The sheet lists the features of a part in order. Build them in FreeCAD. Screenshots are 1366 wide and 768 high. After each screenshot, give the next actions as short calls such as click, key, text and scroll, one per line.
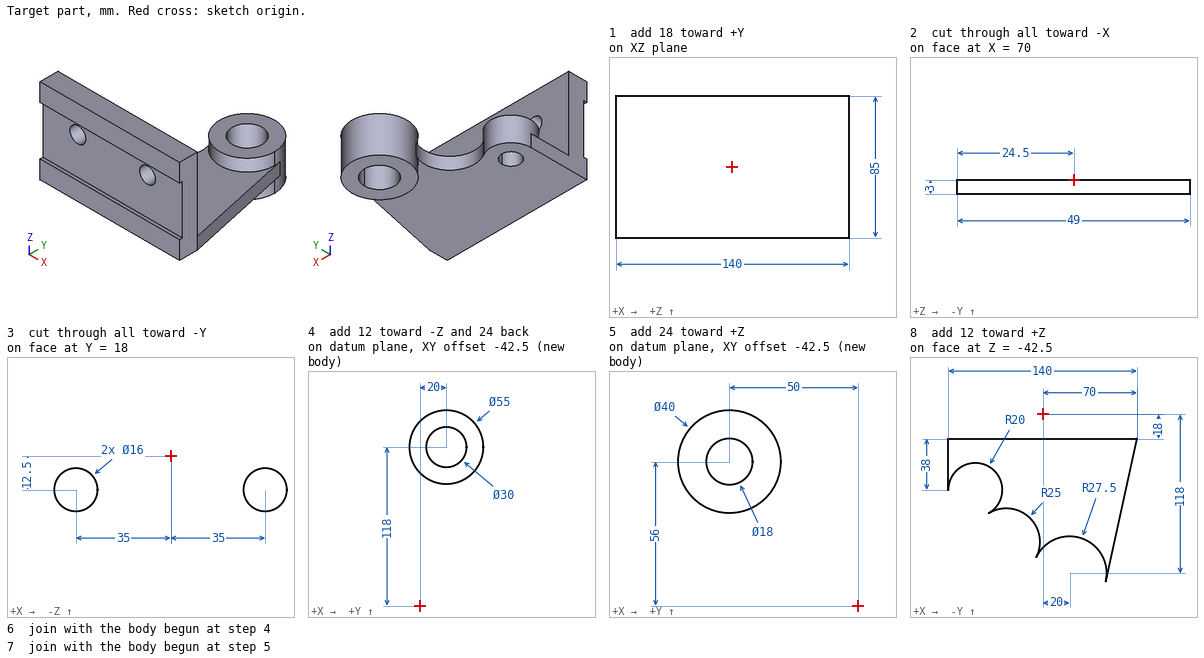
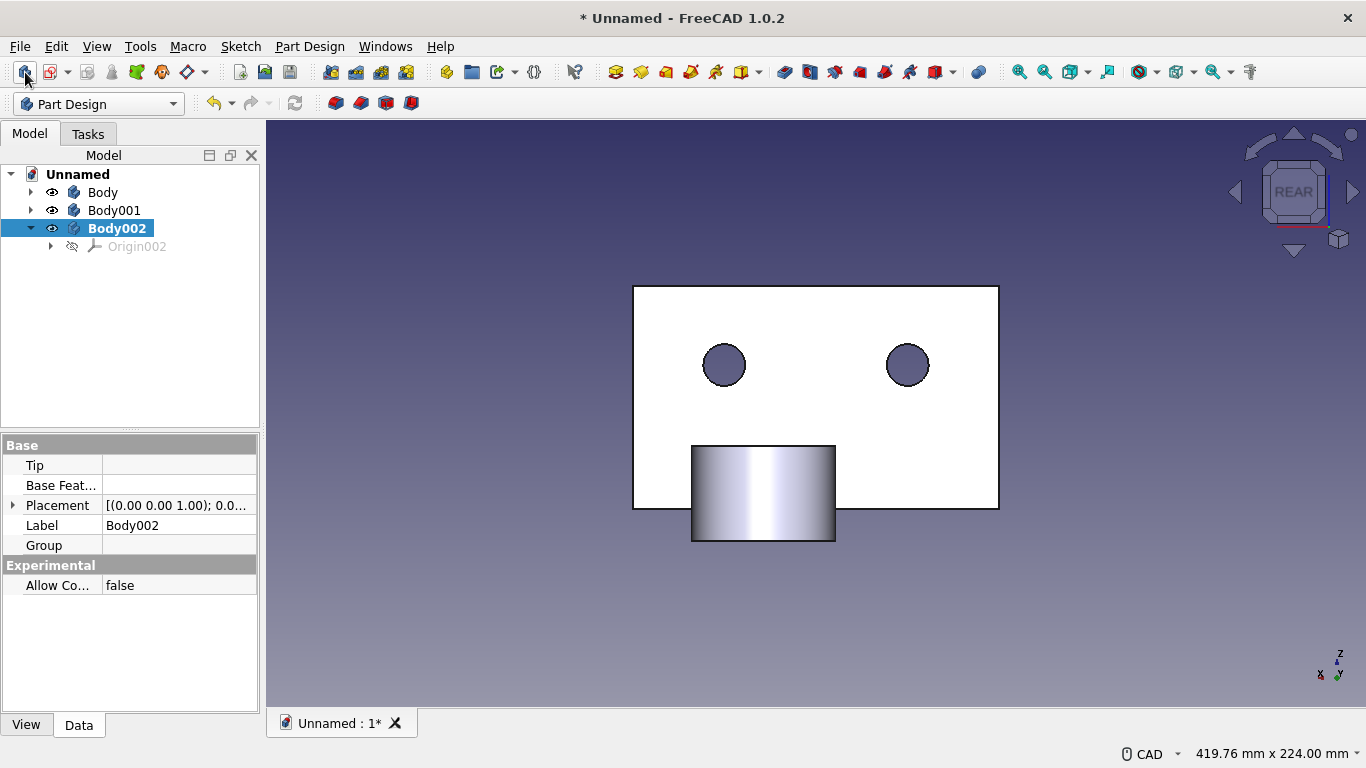
click(51, 246)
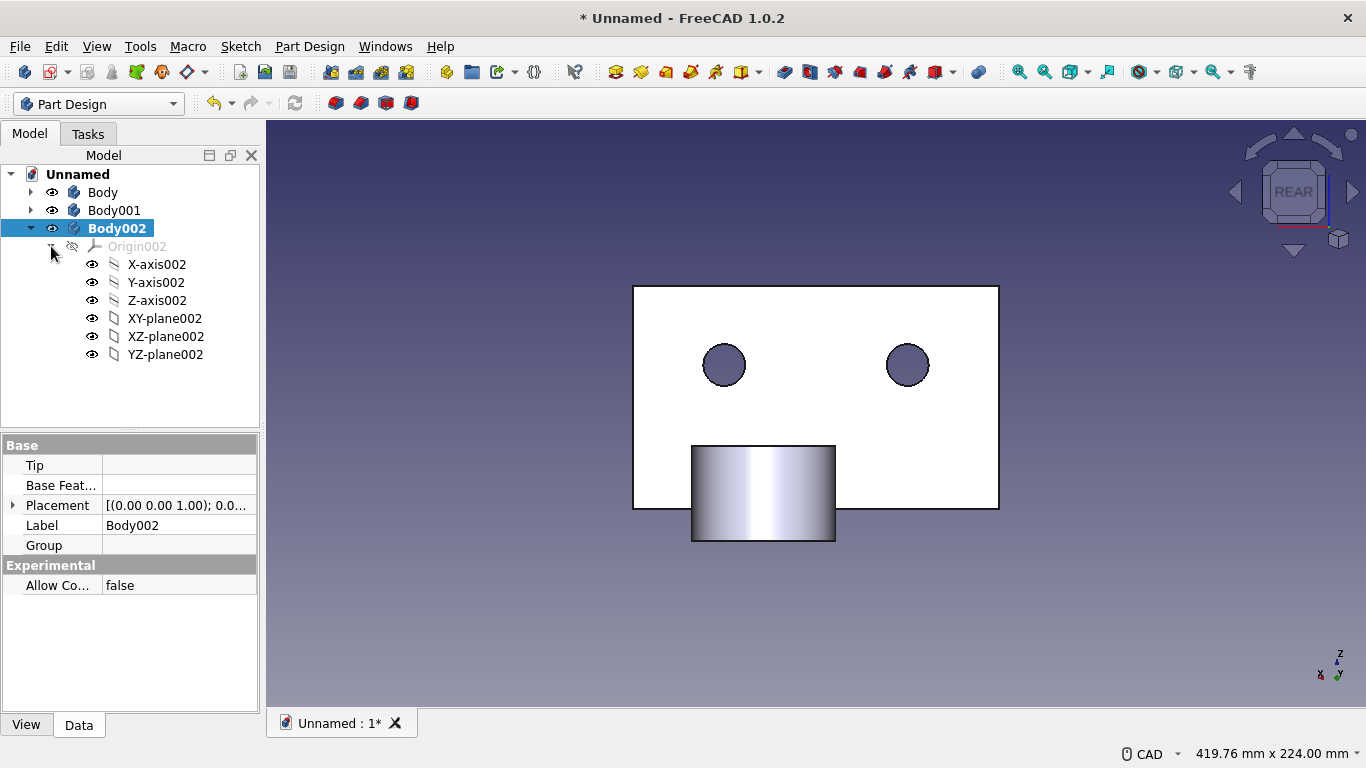
click(137, 318)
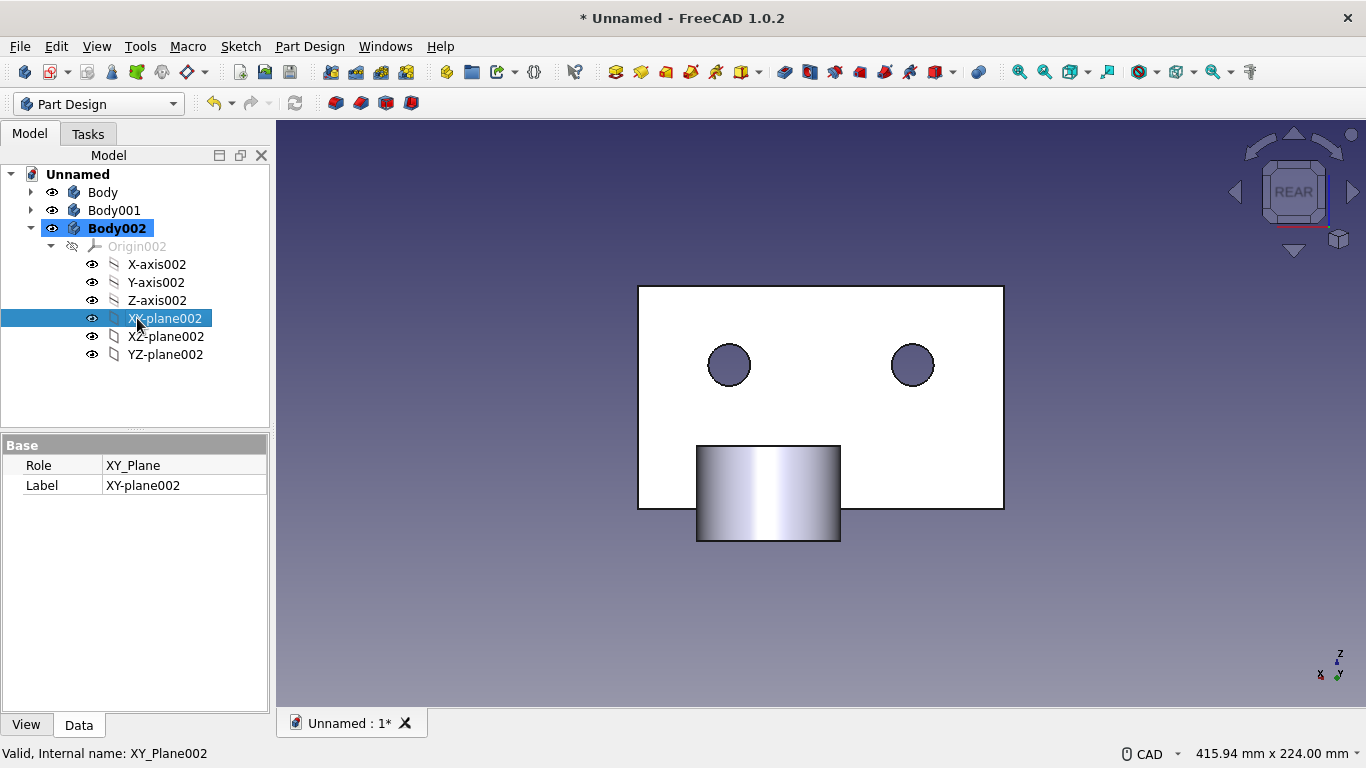
click(186, 72)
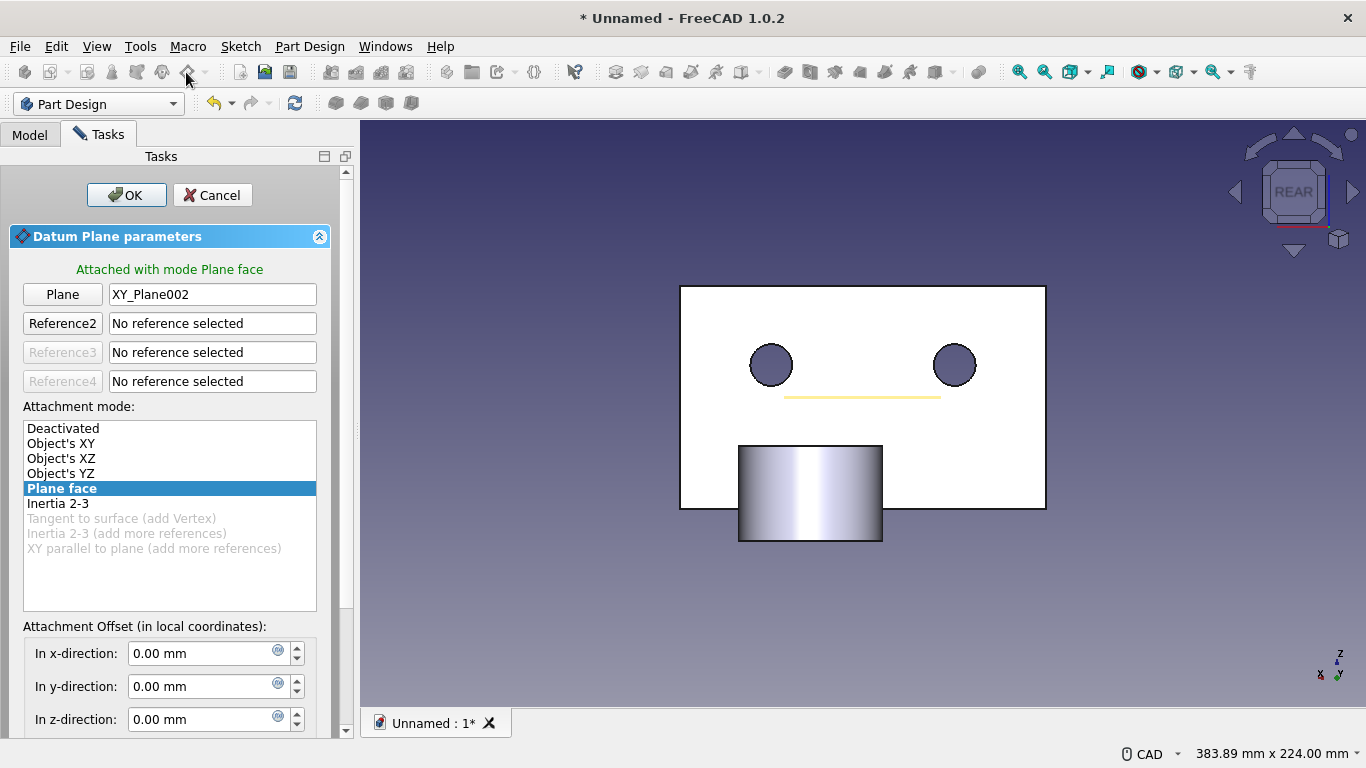
triple_click(210, 720)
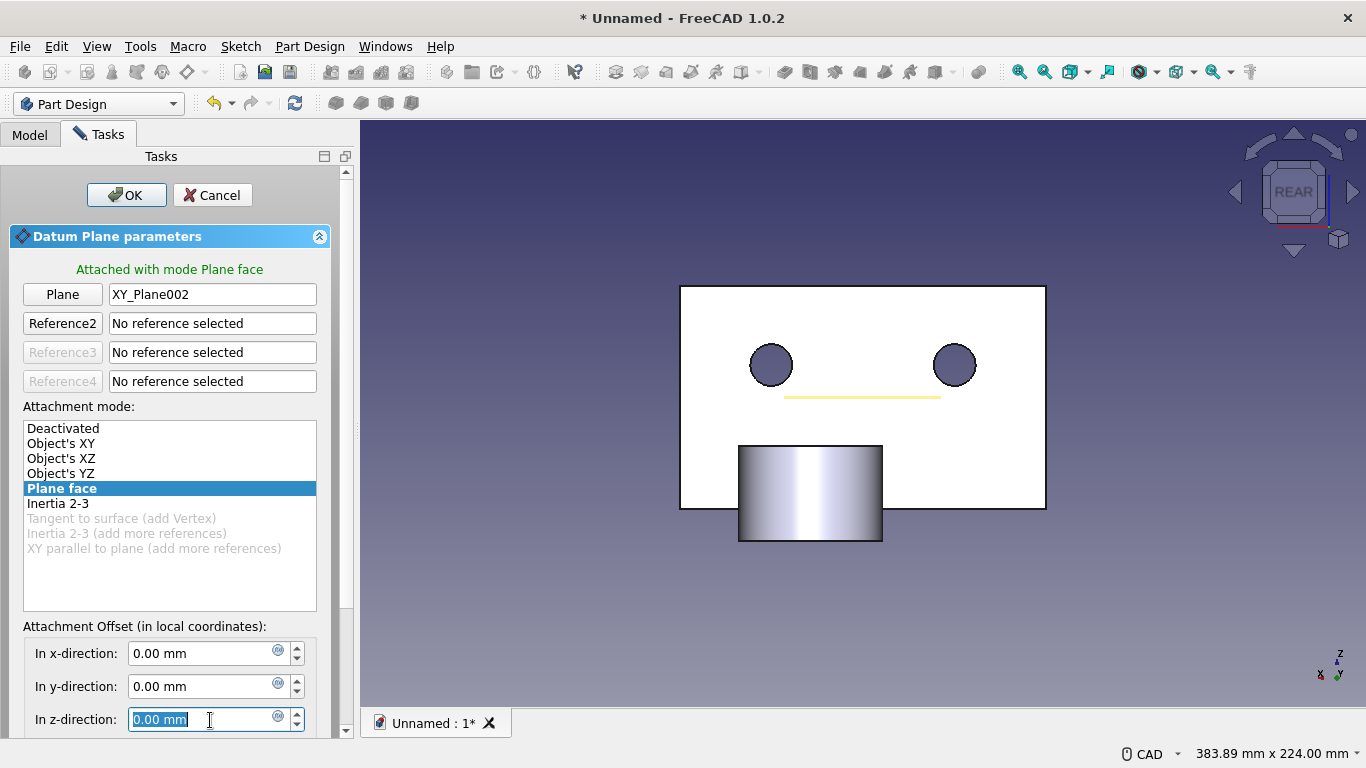
text(-42.5)
key(Tab)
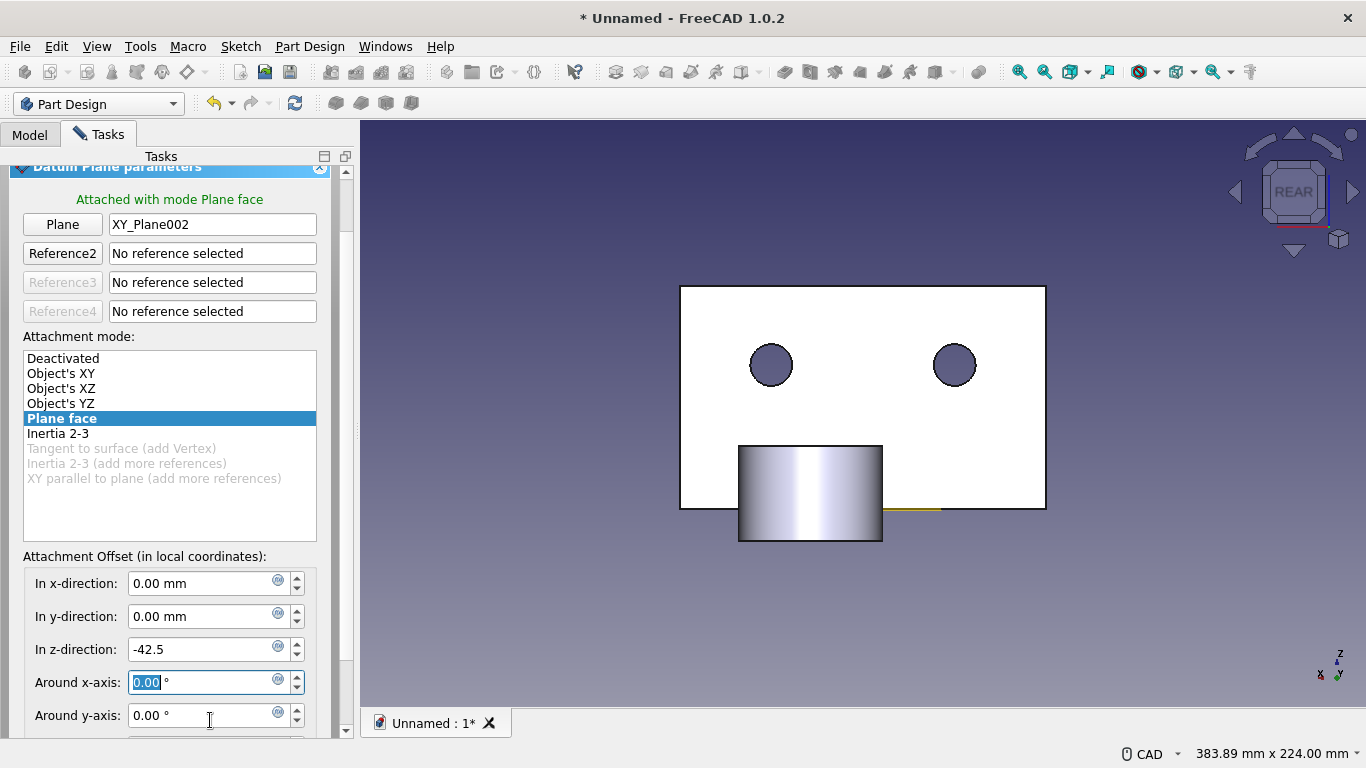
scroll(346, 452, up, 2)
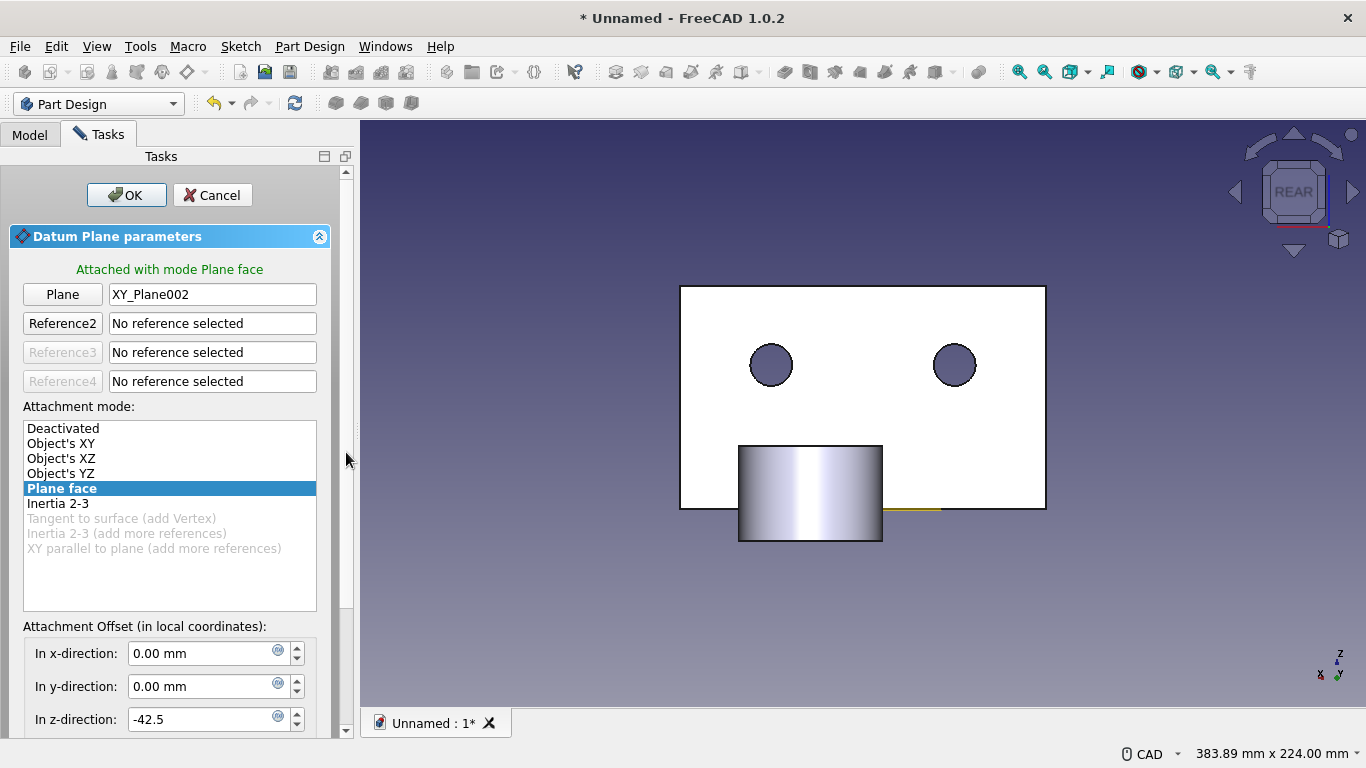
click(127, 195)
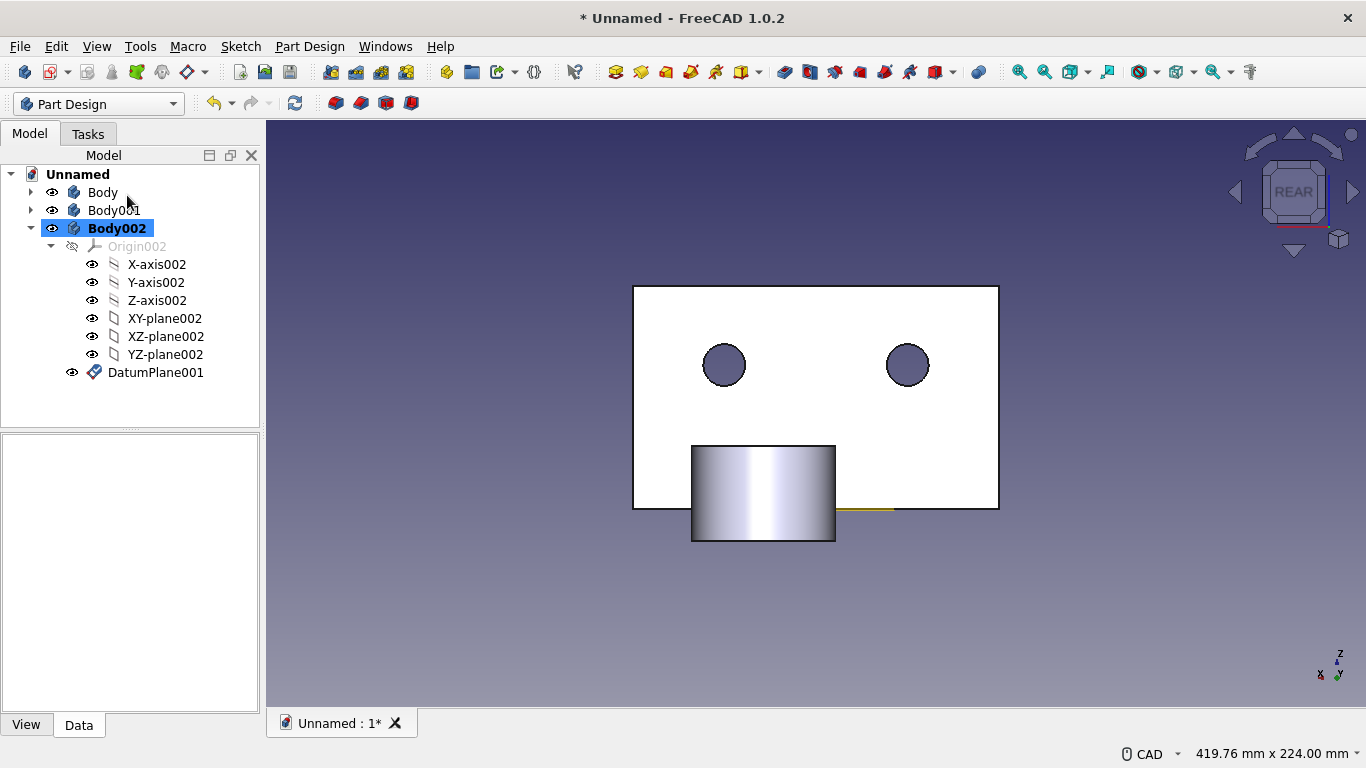
click(117, 372)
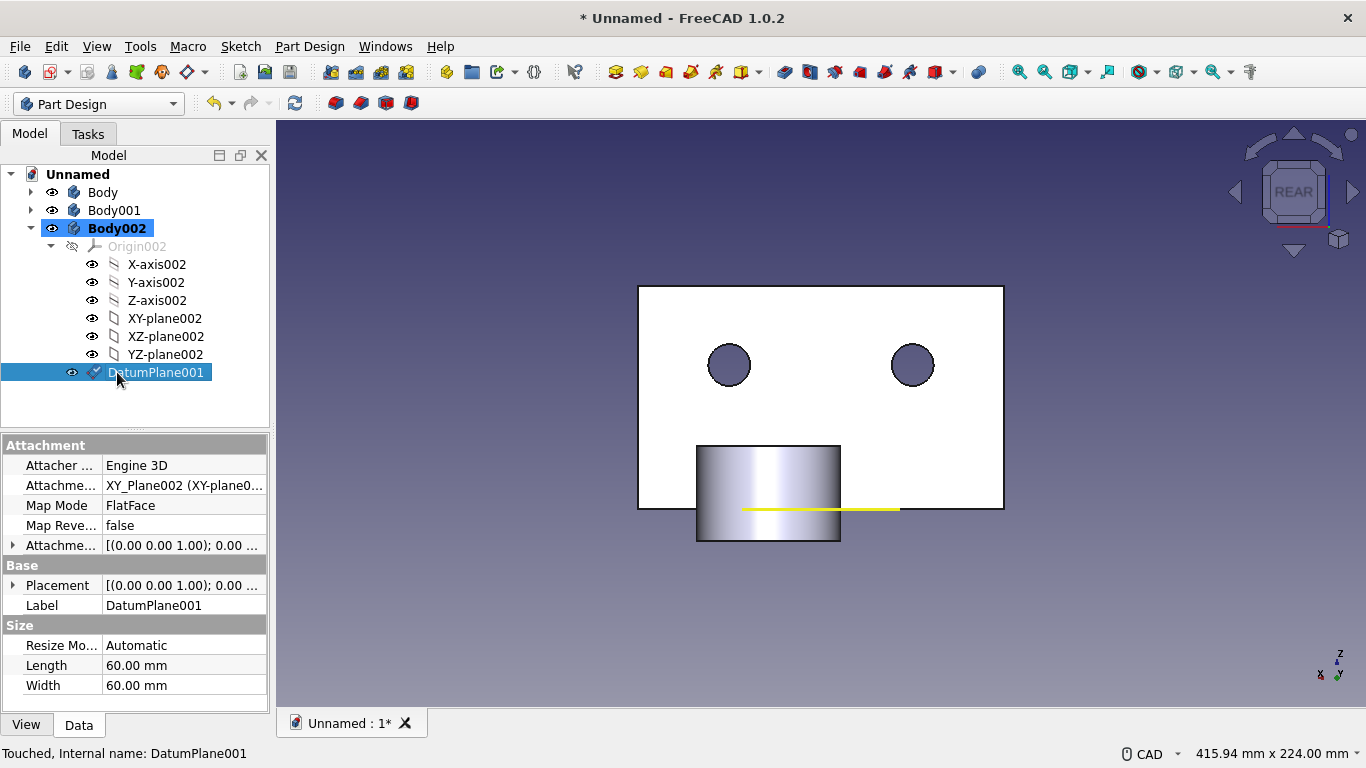
click(50, 72)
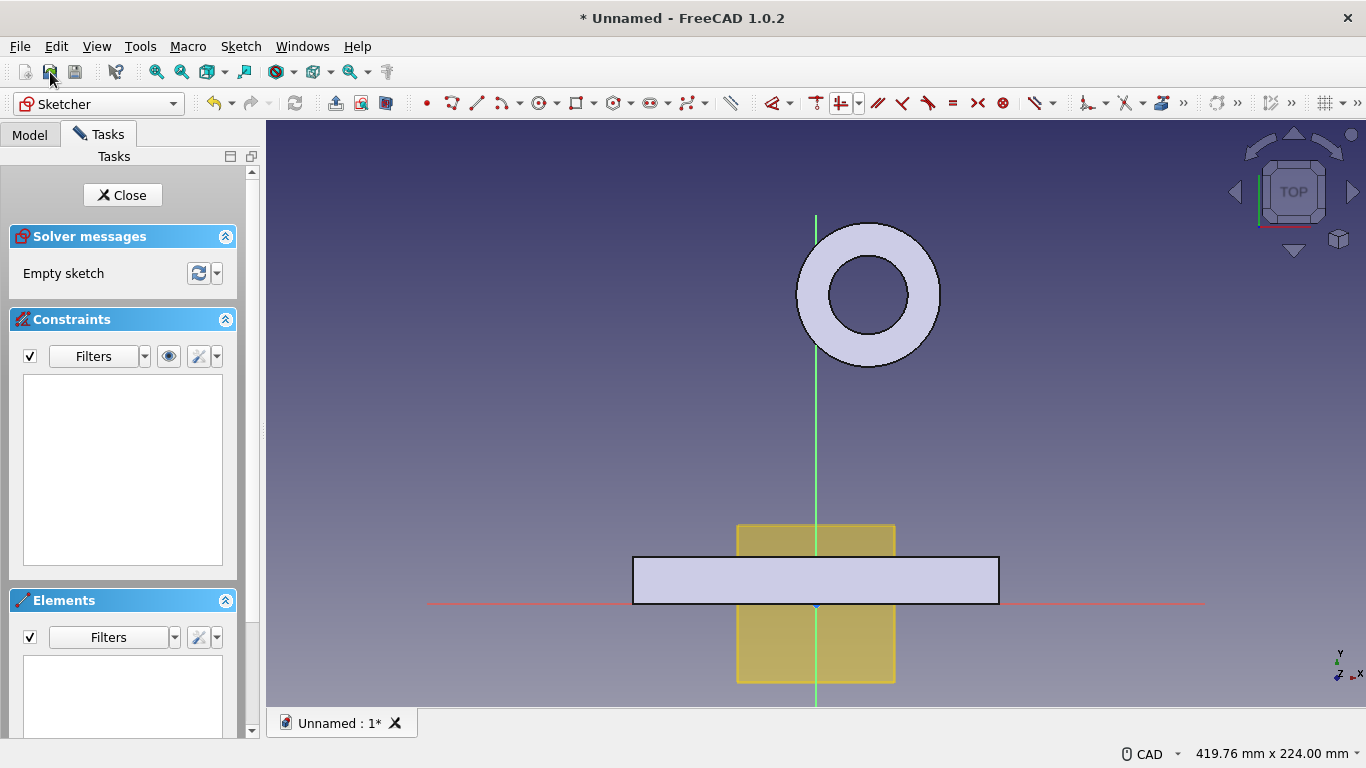
scroll(696, 615, up, 3)